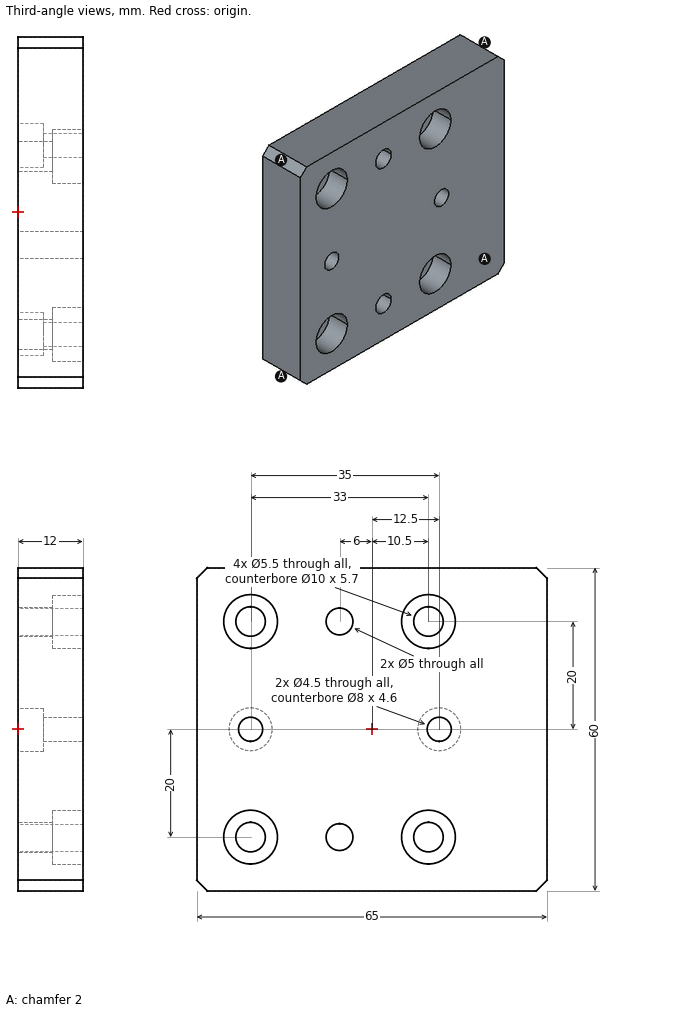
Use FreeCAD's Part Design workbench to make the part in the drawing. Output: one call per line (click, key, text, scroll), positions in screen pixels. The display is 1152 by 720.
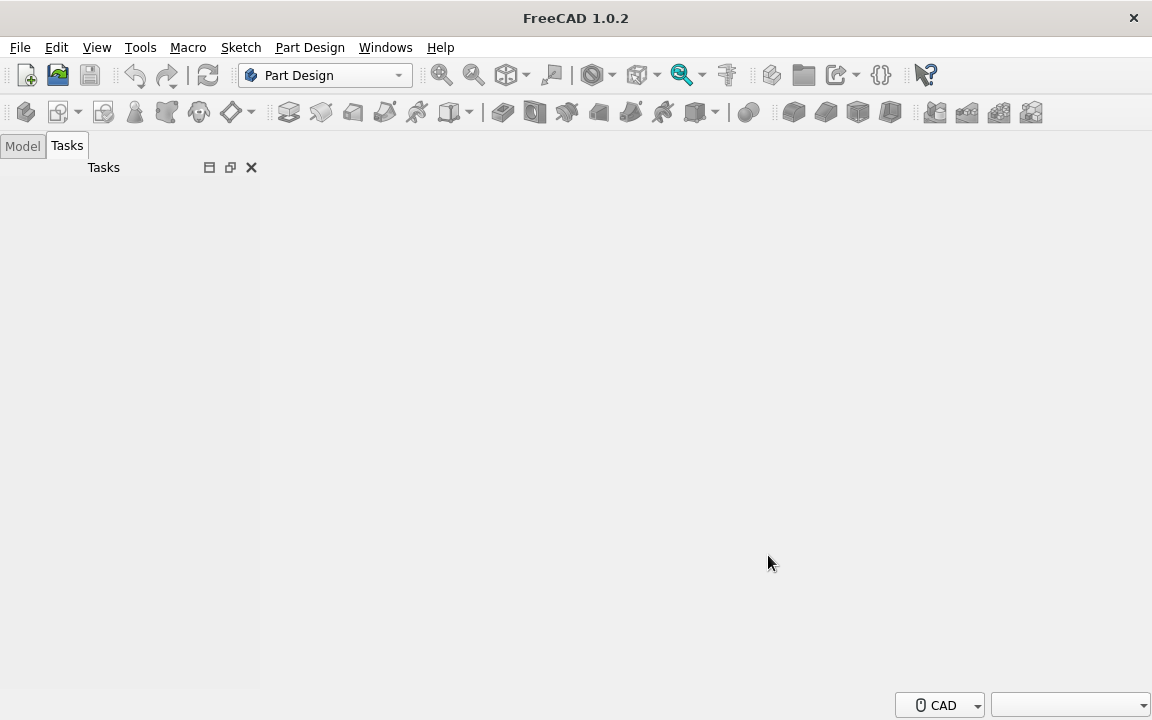
click(26, 76)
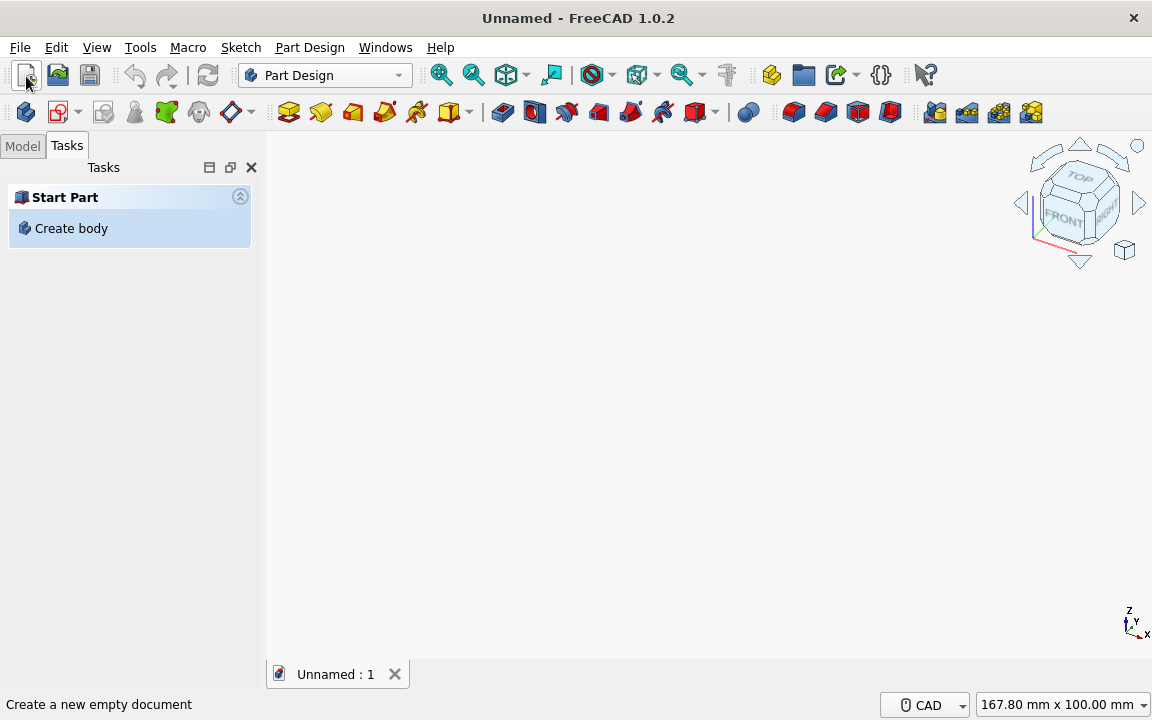
click(58, 112)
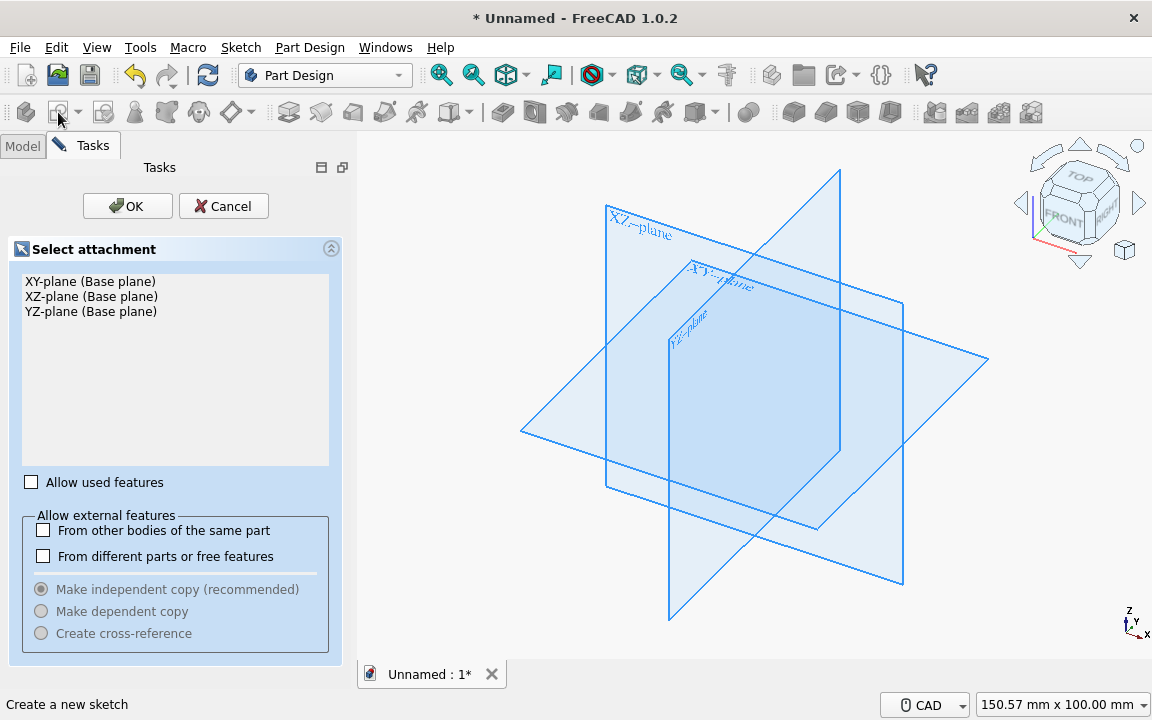
click(82, 312)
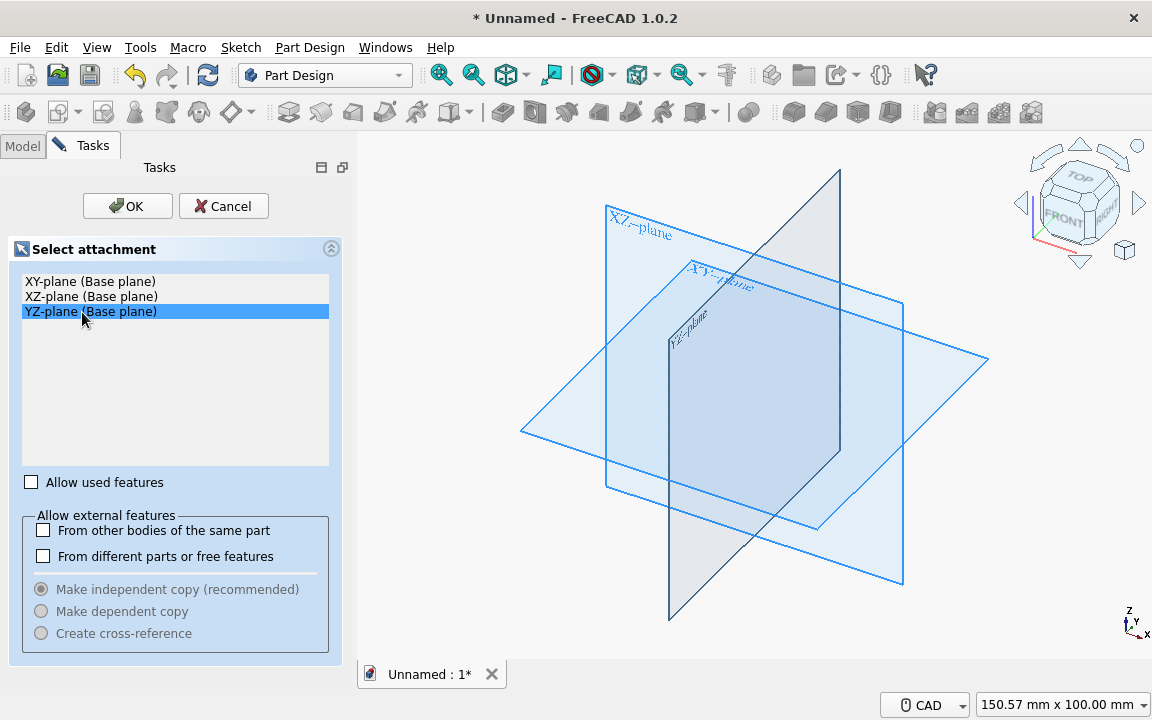
click(128, 206)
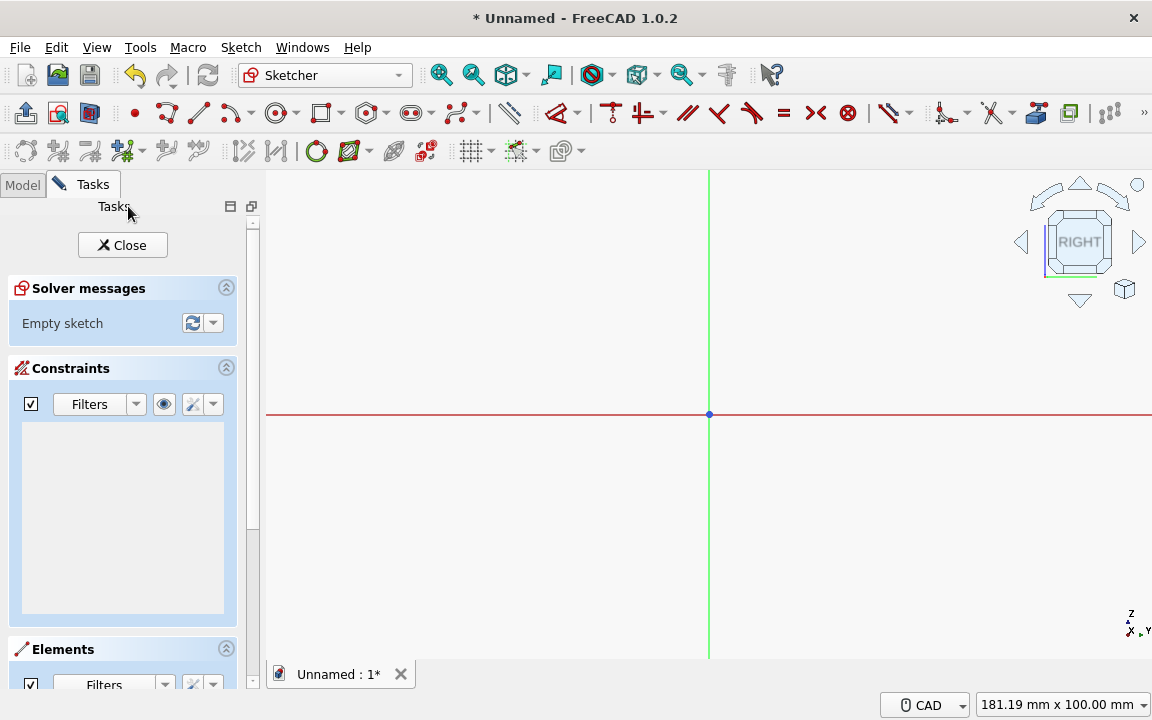
click(344, 114)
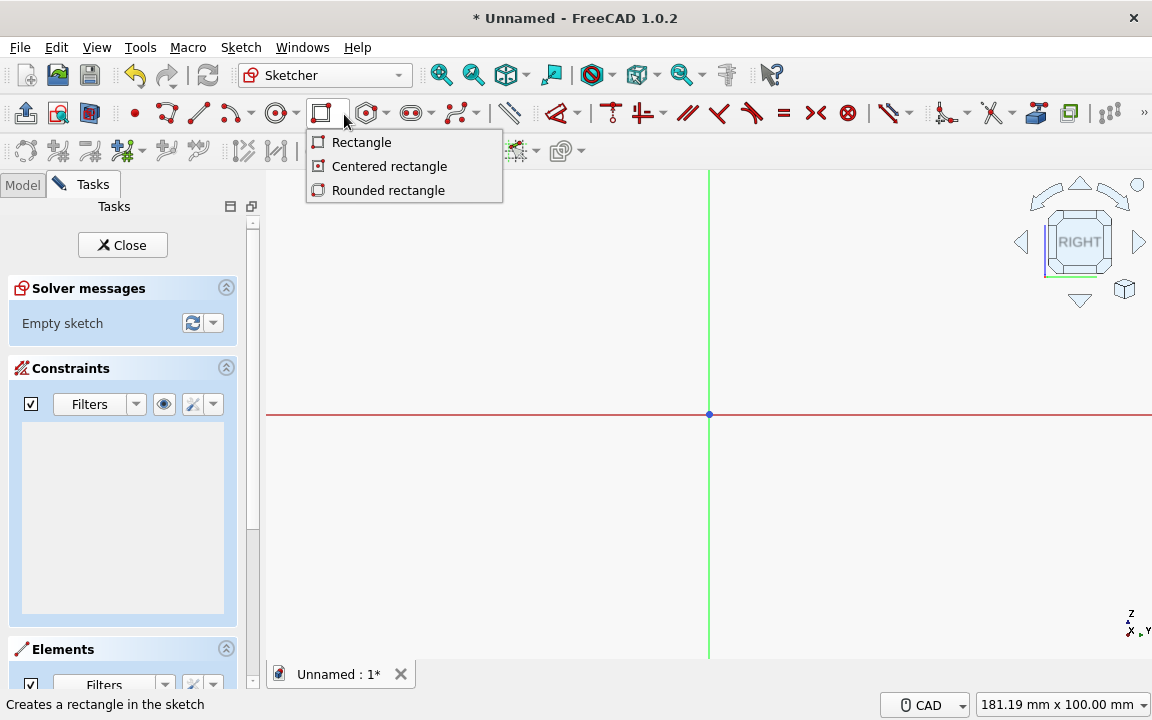
click(404, 166)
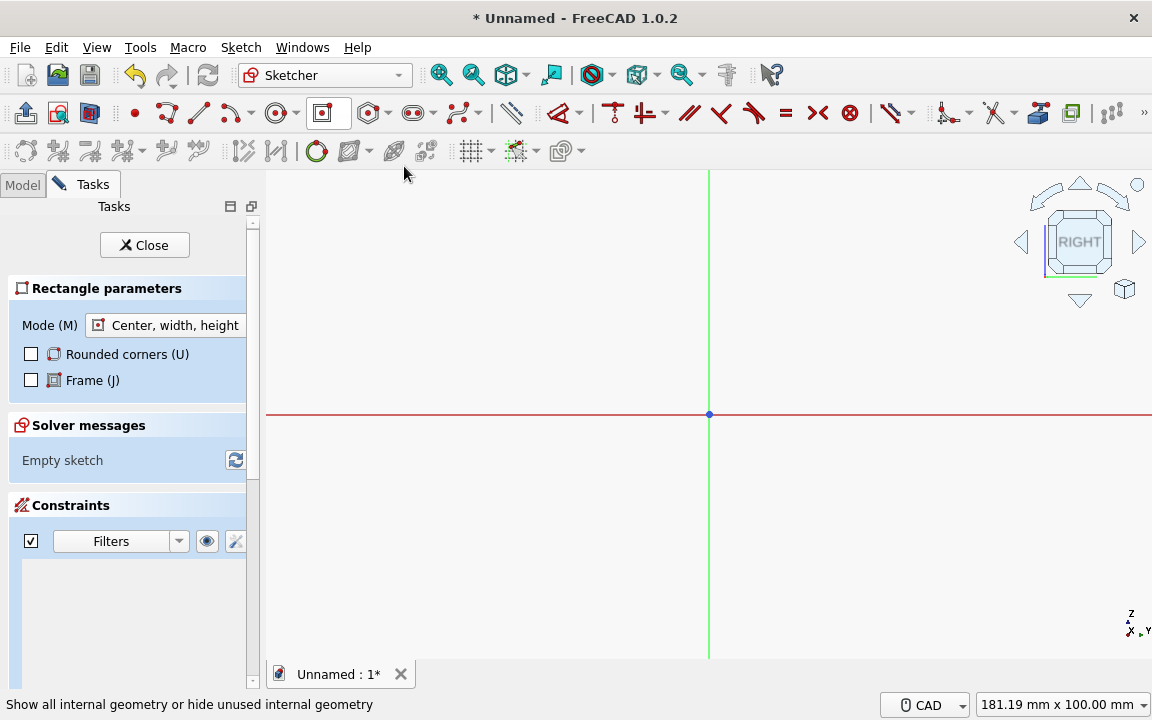
click(709, 414)
click(868, 268)
key(Escape)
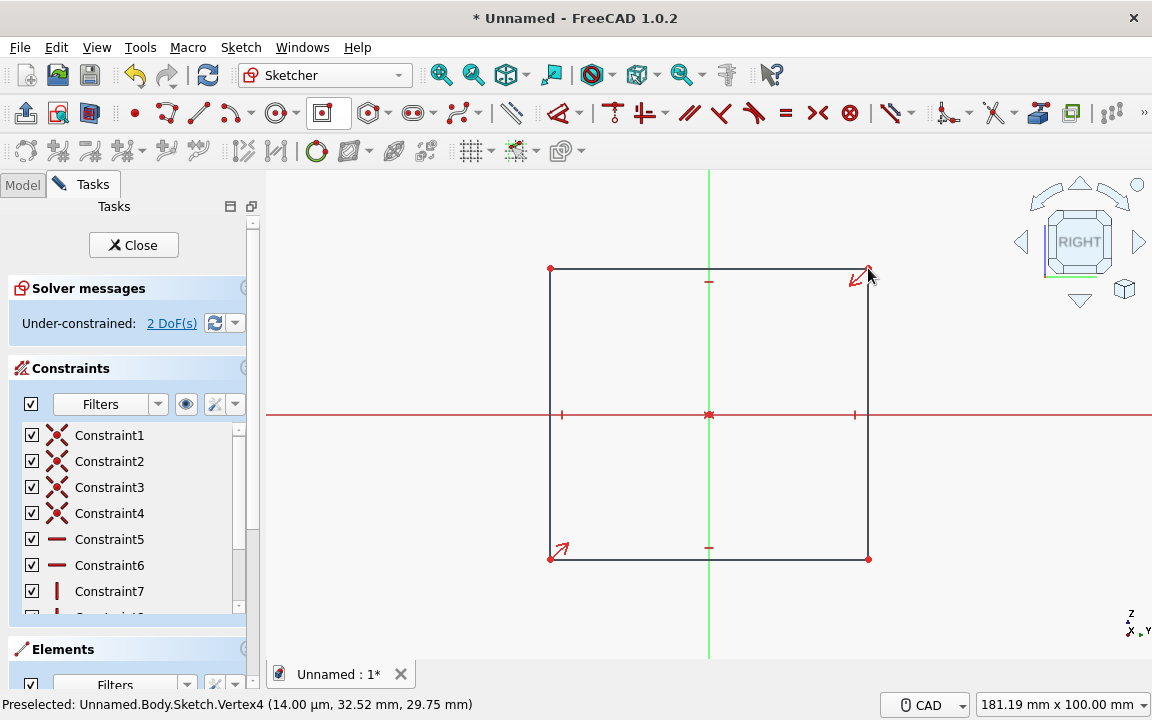
click(558, 114)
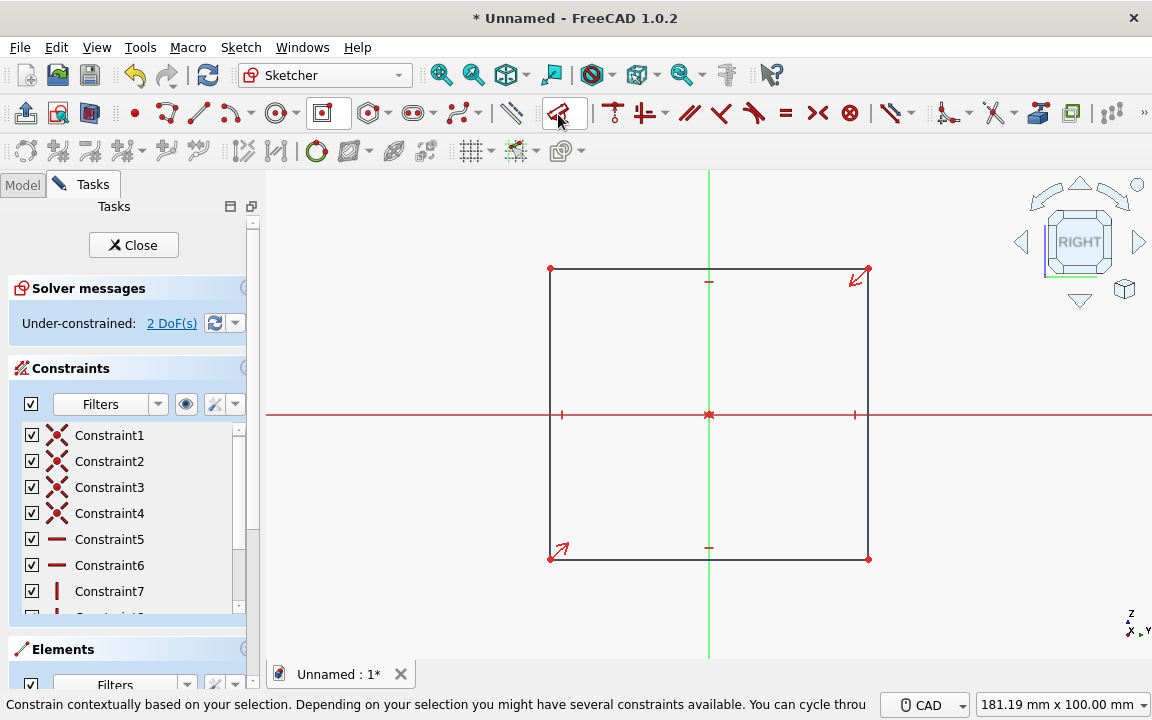
click(645, 560)
click(636, 594)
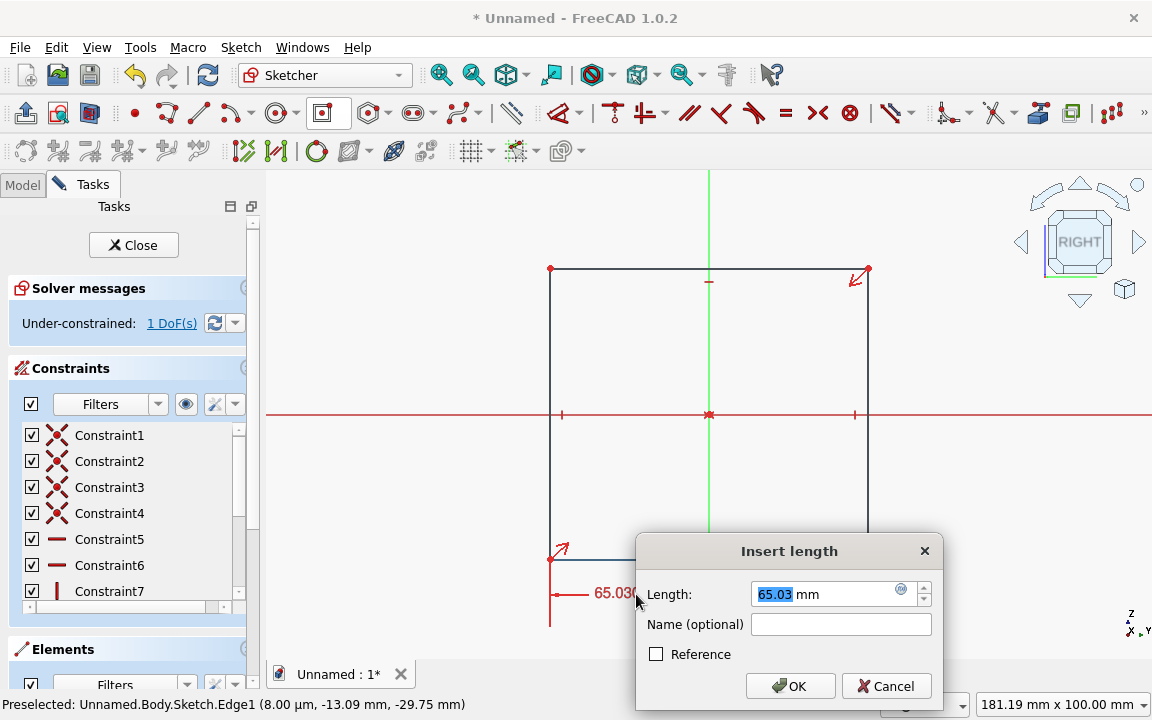
text(65)
key(Return)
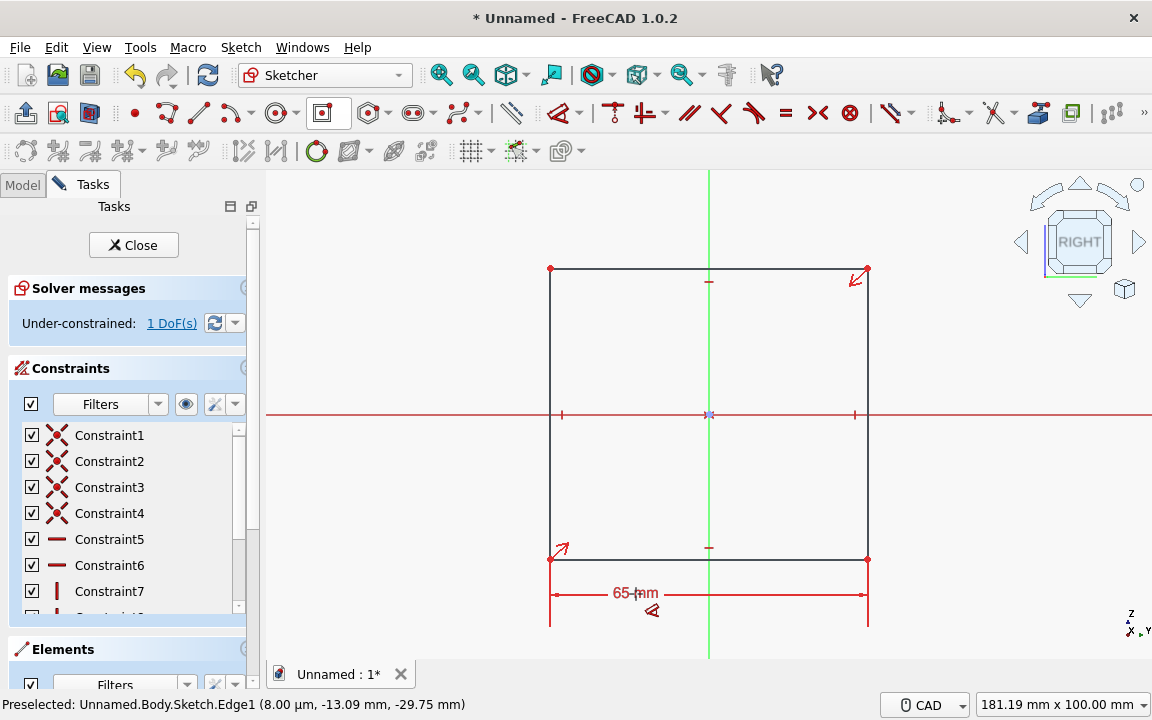
click(868, 473)
click(902, 348)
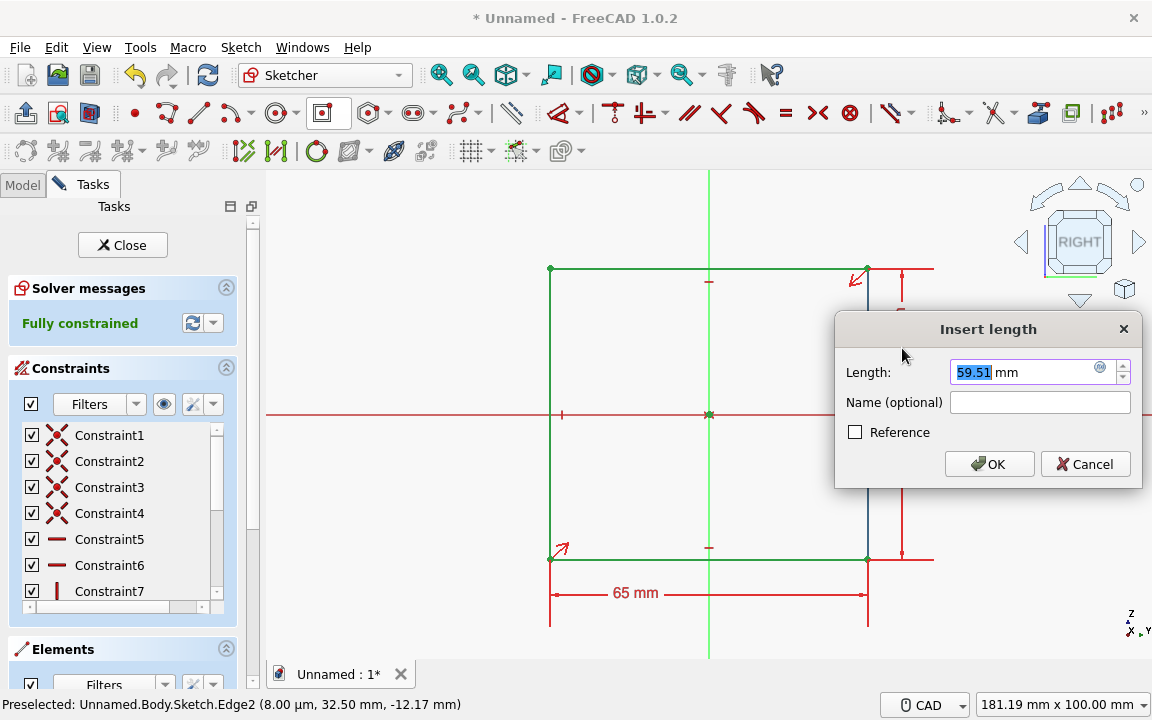
text(60)
key(Return)
key(Escape)